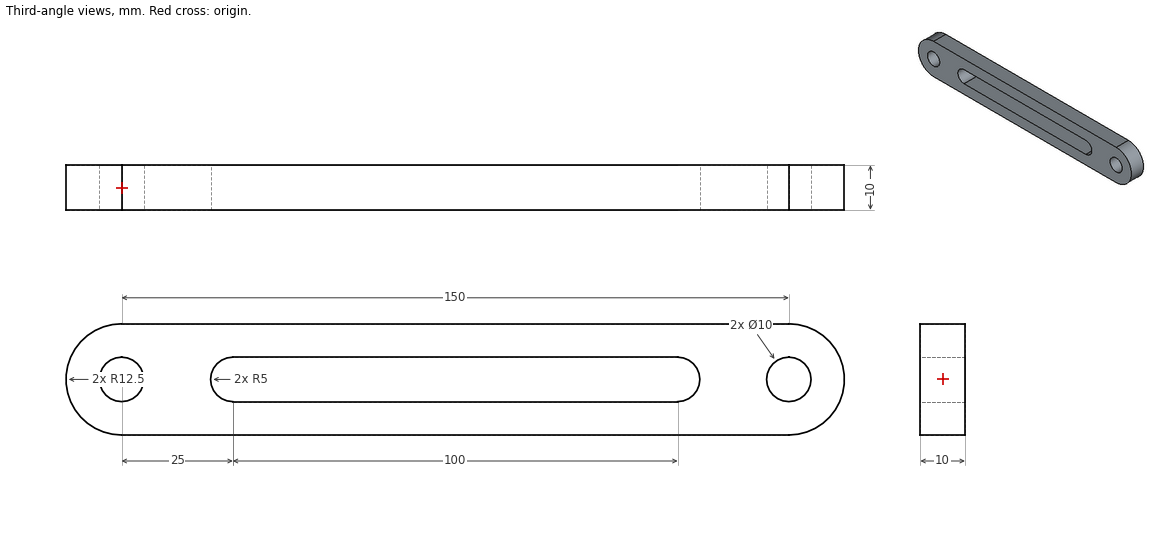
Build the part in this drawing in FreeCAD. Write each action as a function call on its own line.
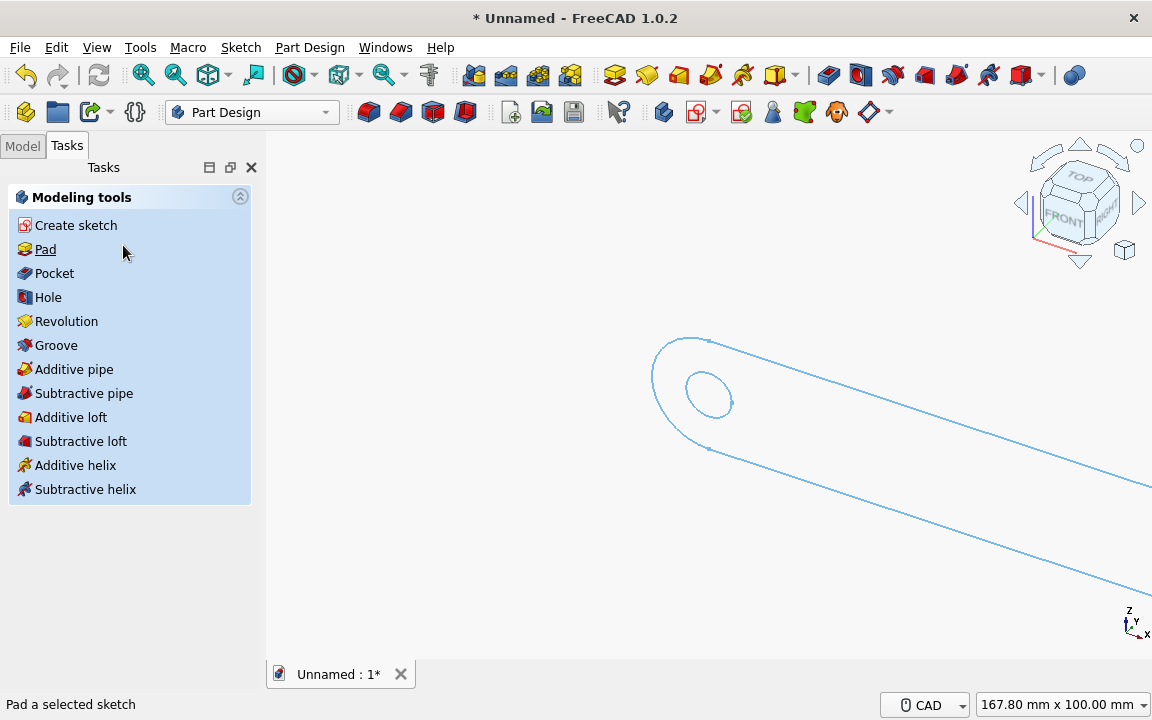
click(616, 76)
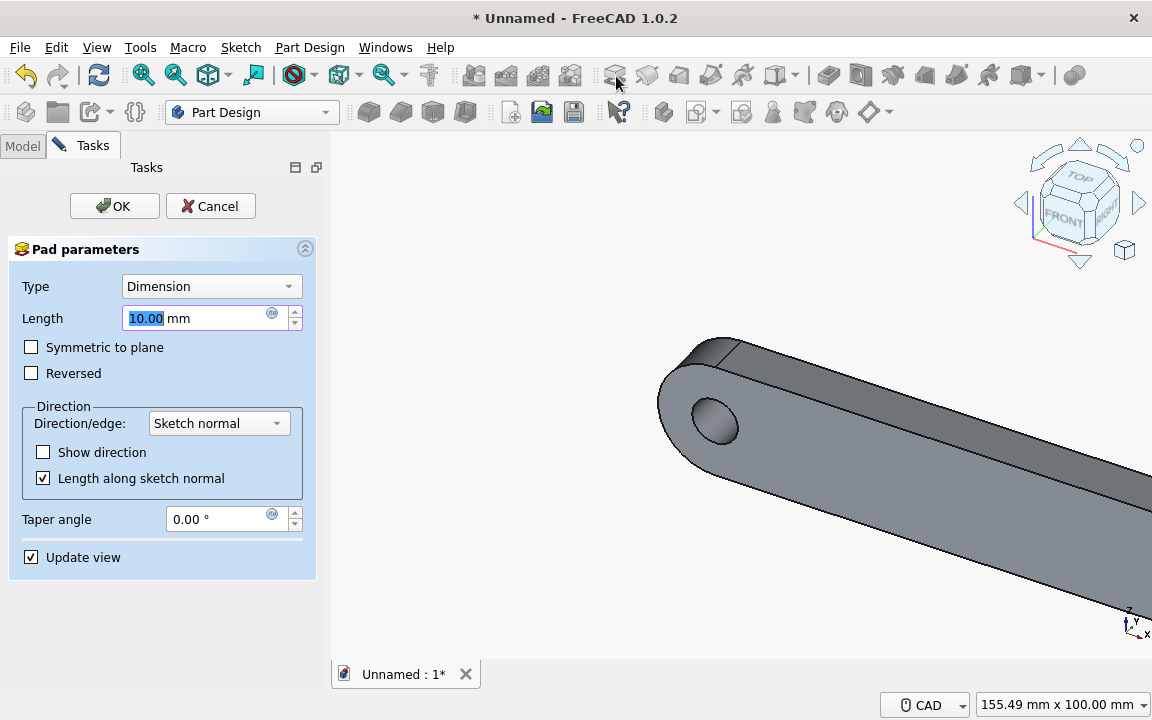
text(10)
key(Tab)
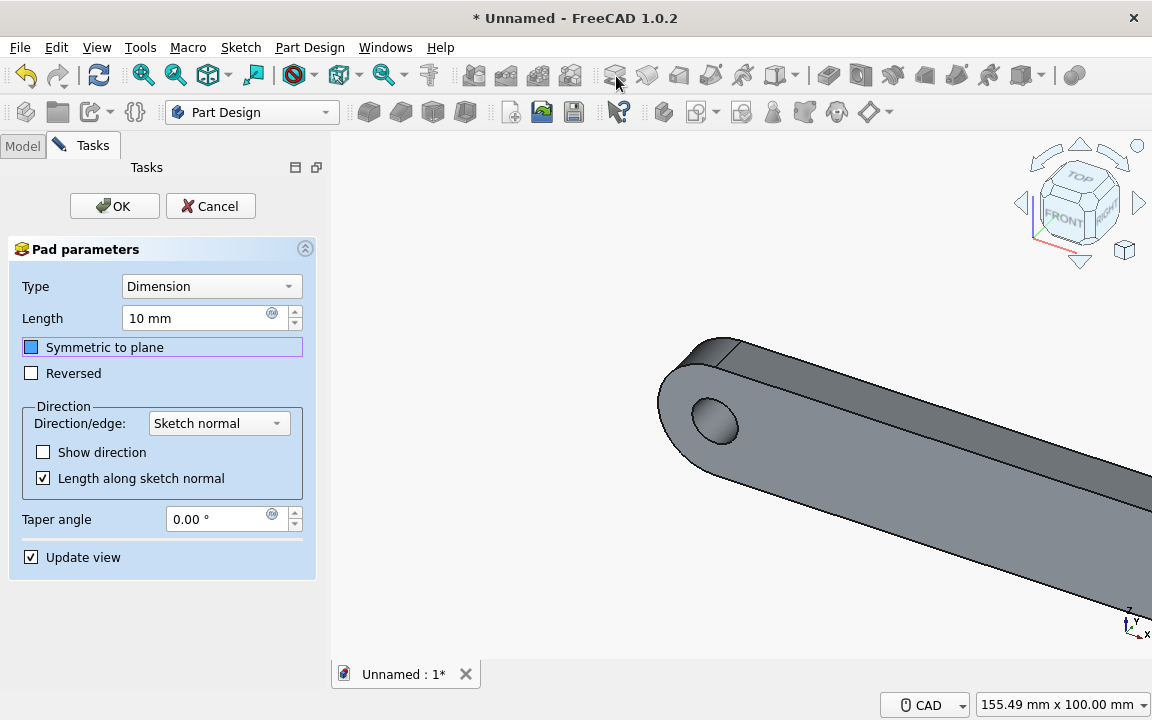
click(30, 347)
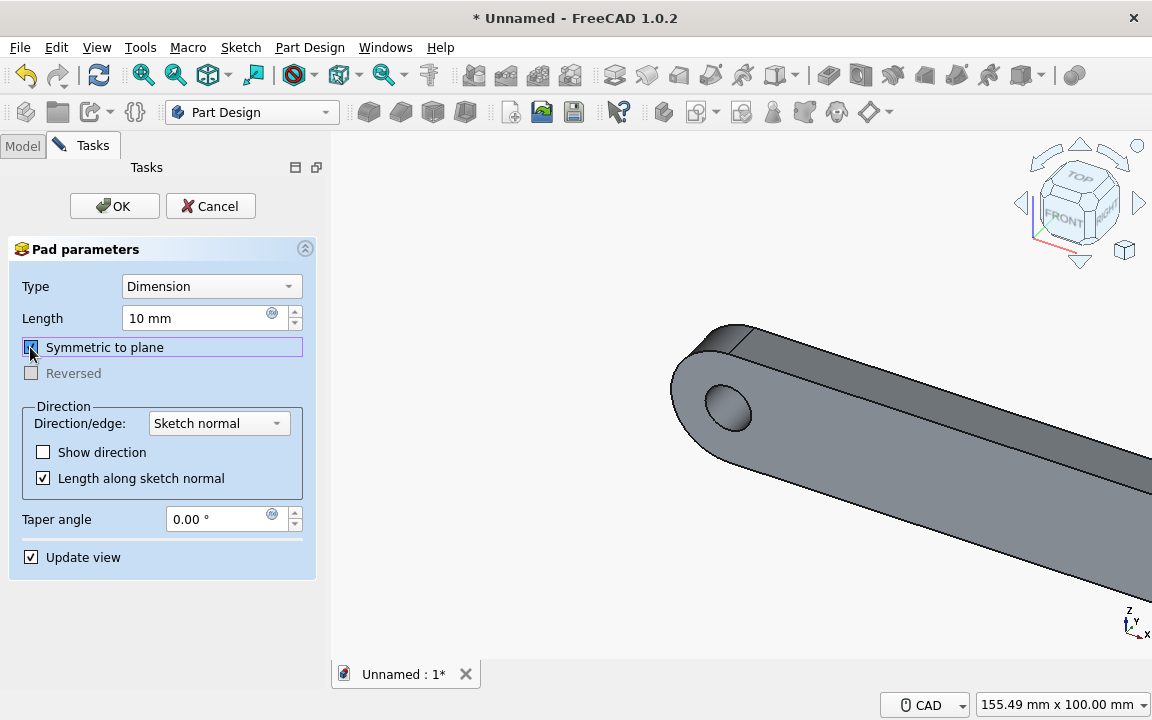
click(115, 206)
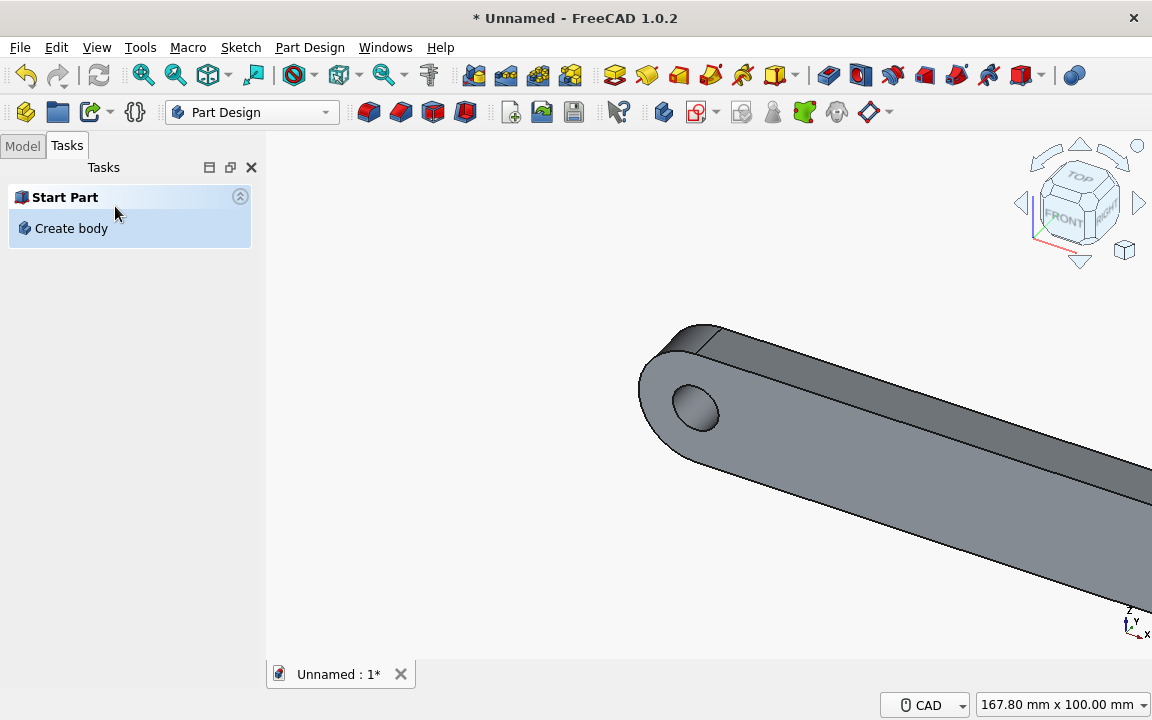
click(144, 76)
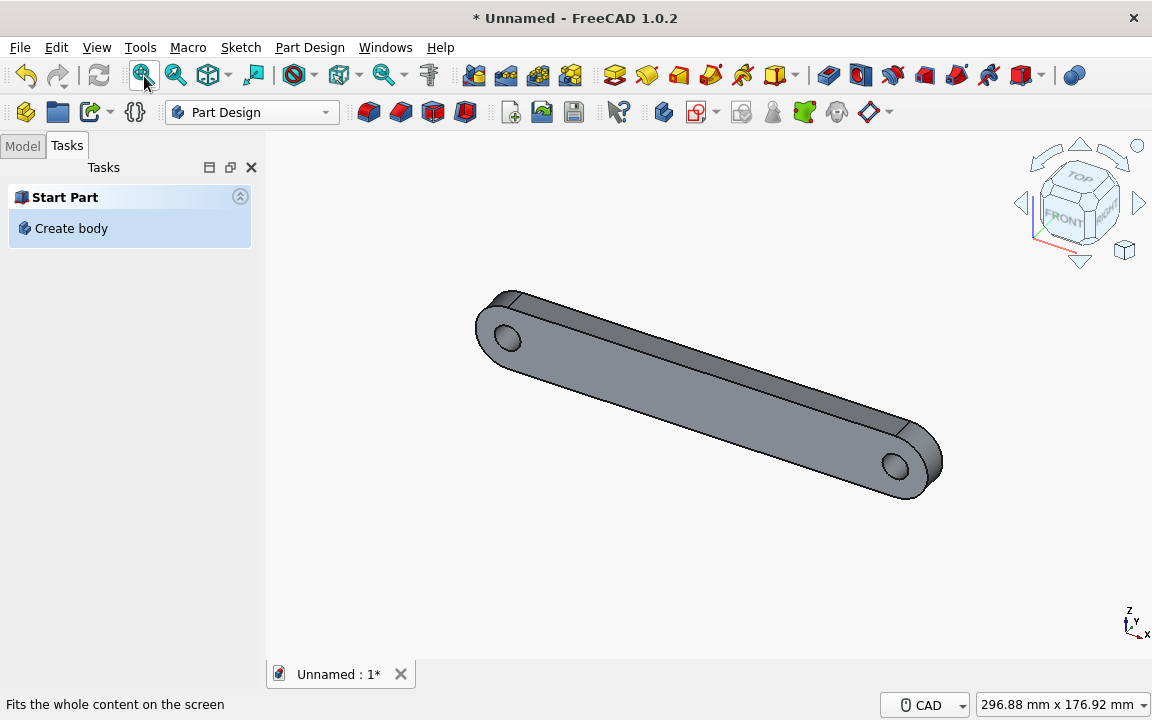
key(4)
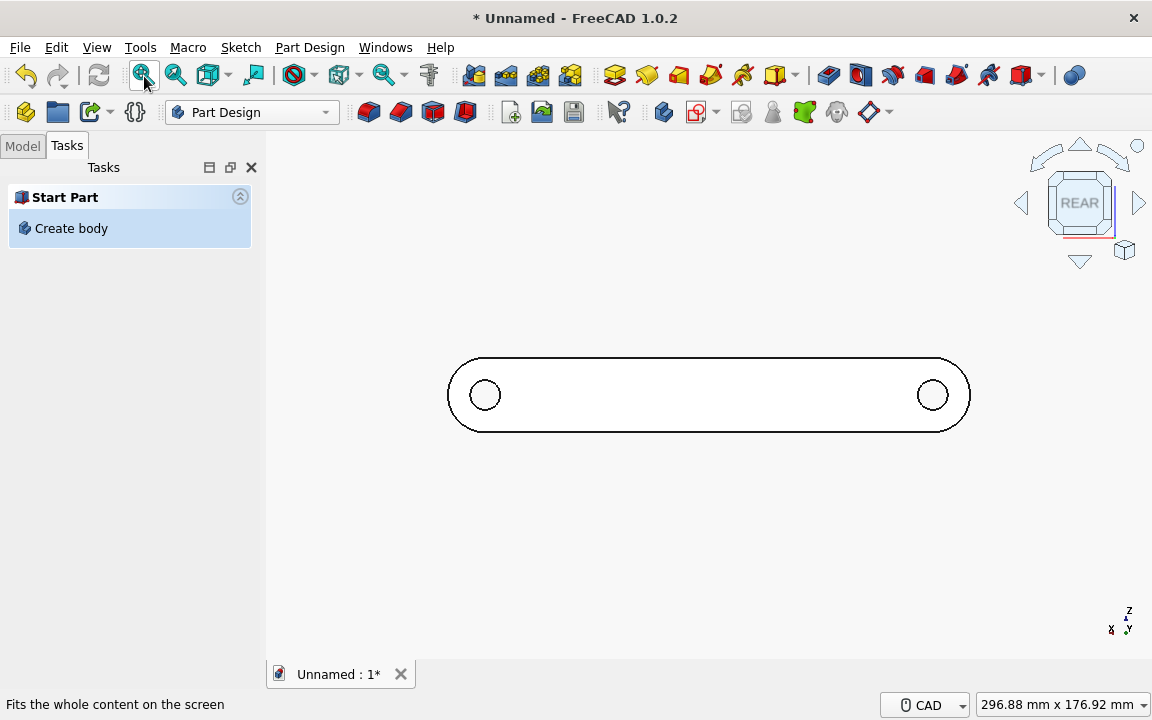
click(560, 394)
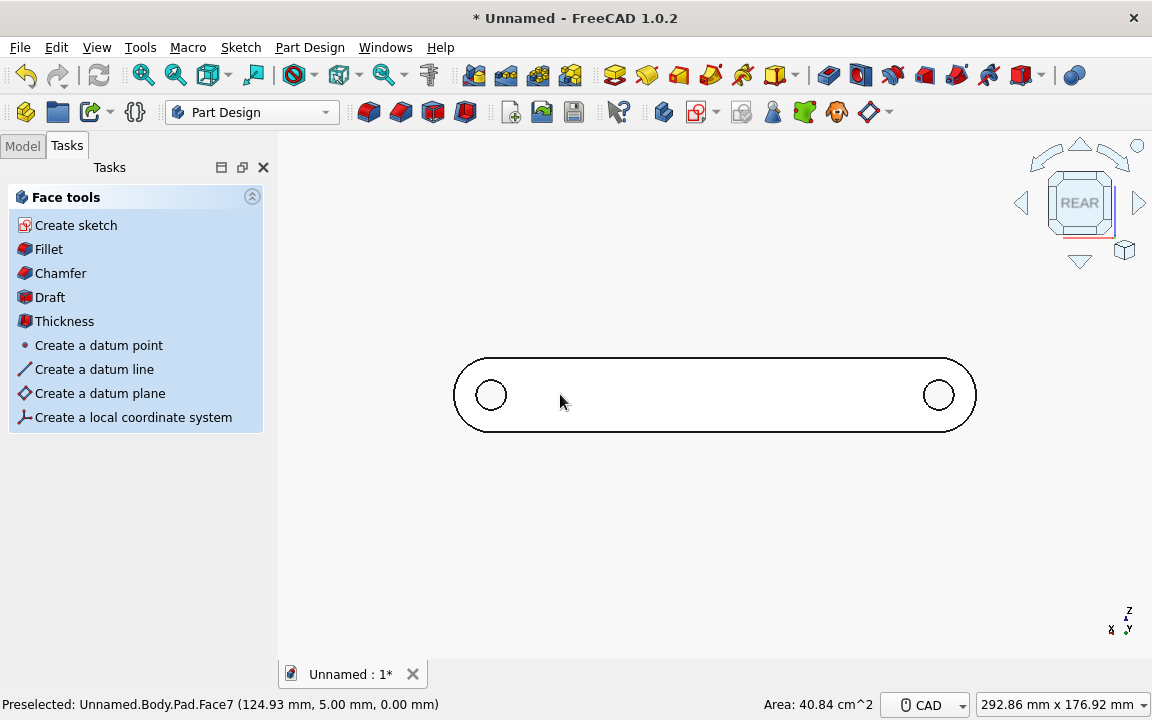
click(696, 112)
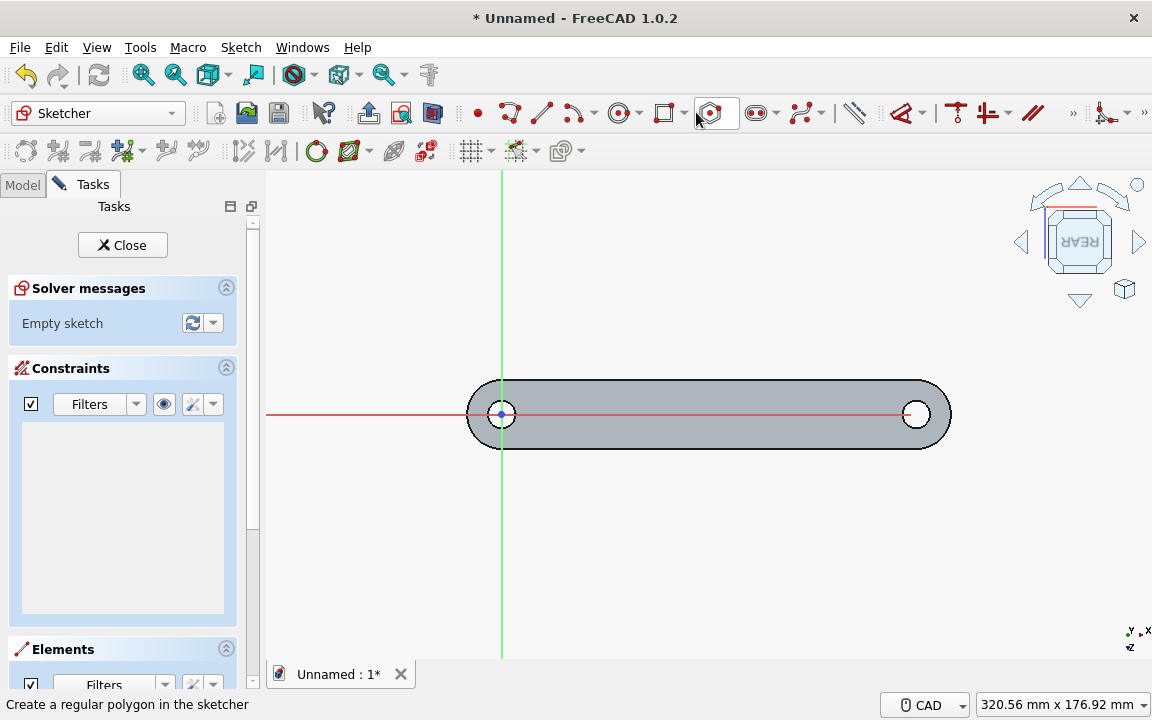
scroll(764, 415, up, 2)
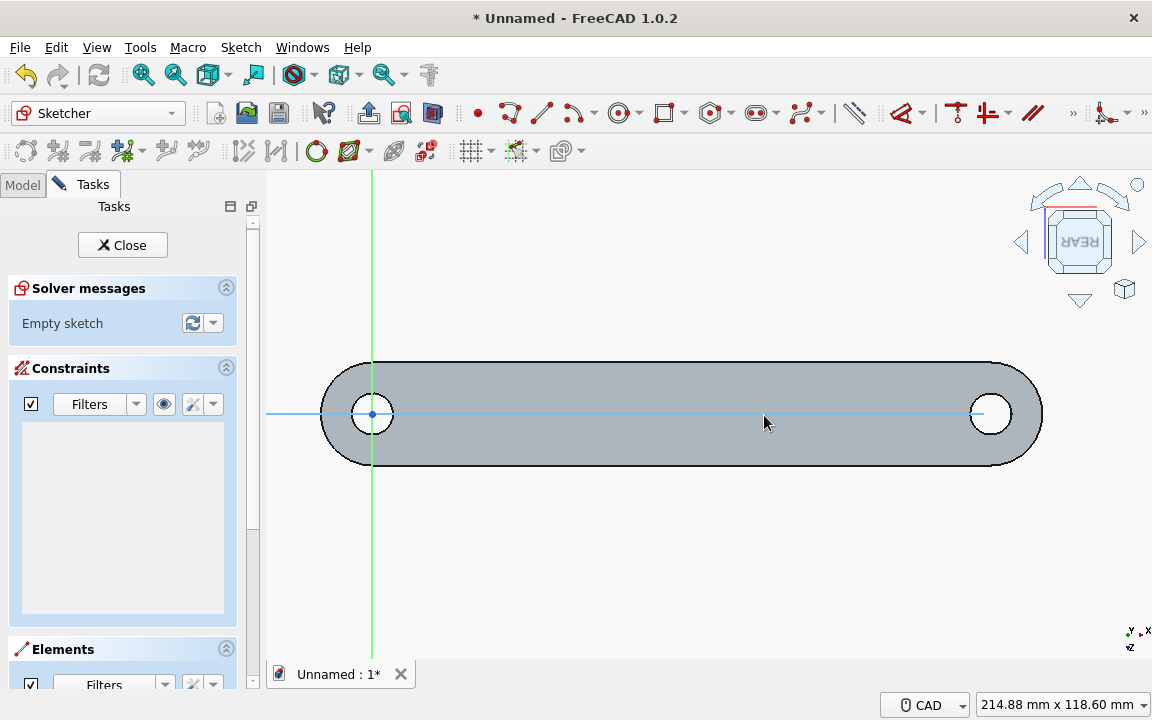
click(756, 114)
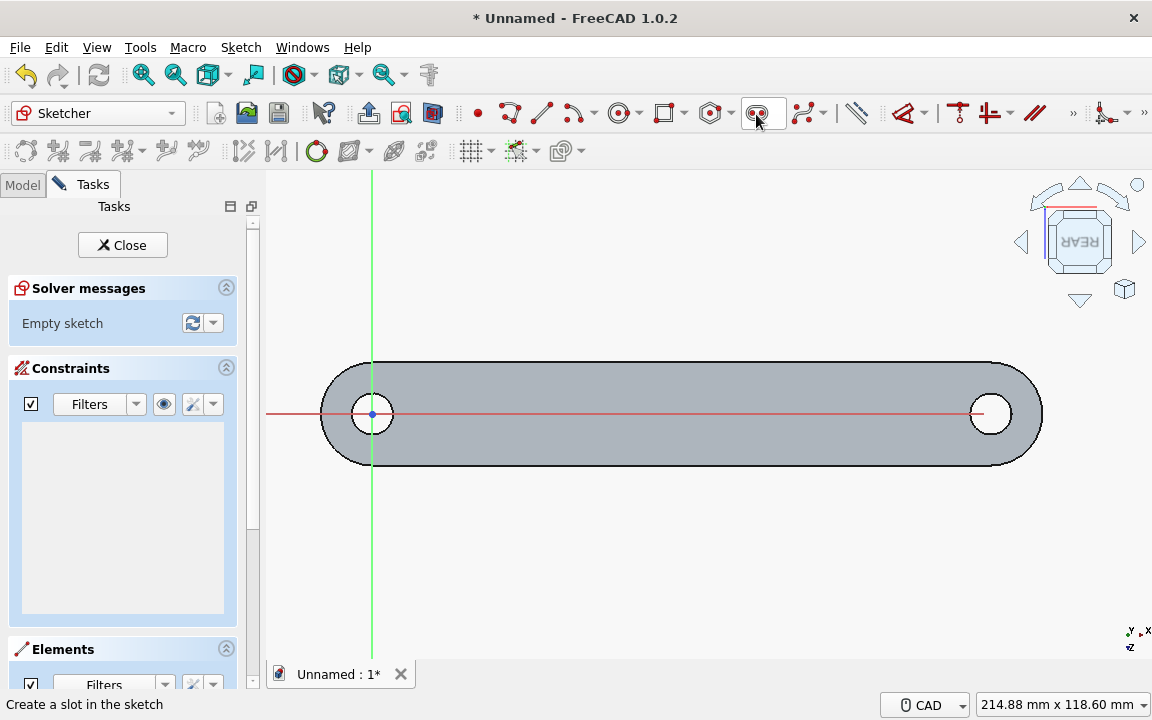
click(476, 414)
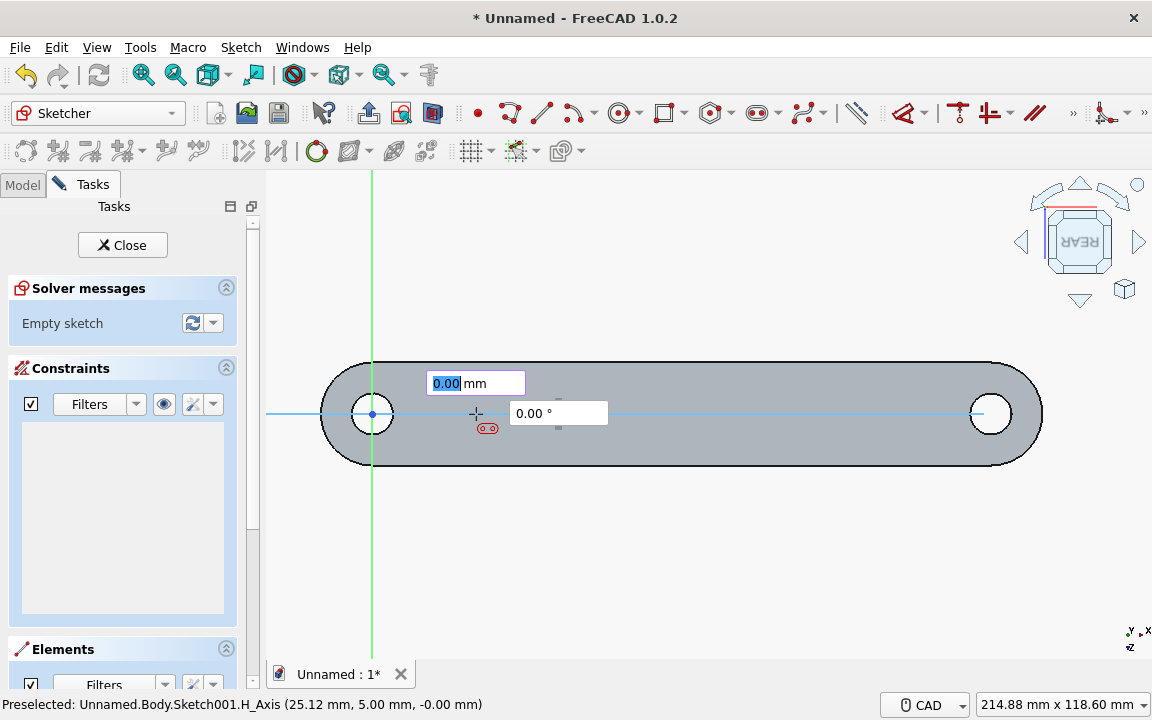
click(888, 405)